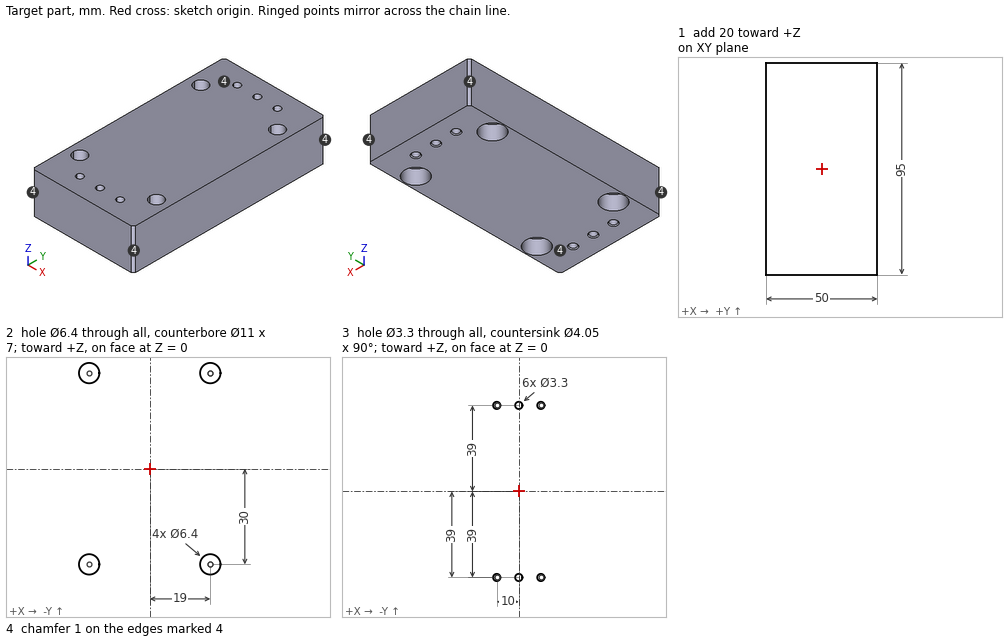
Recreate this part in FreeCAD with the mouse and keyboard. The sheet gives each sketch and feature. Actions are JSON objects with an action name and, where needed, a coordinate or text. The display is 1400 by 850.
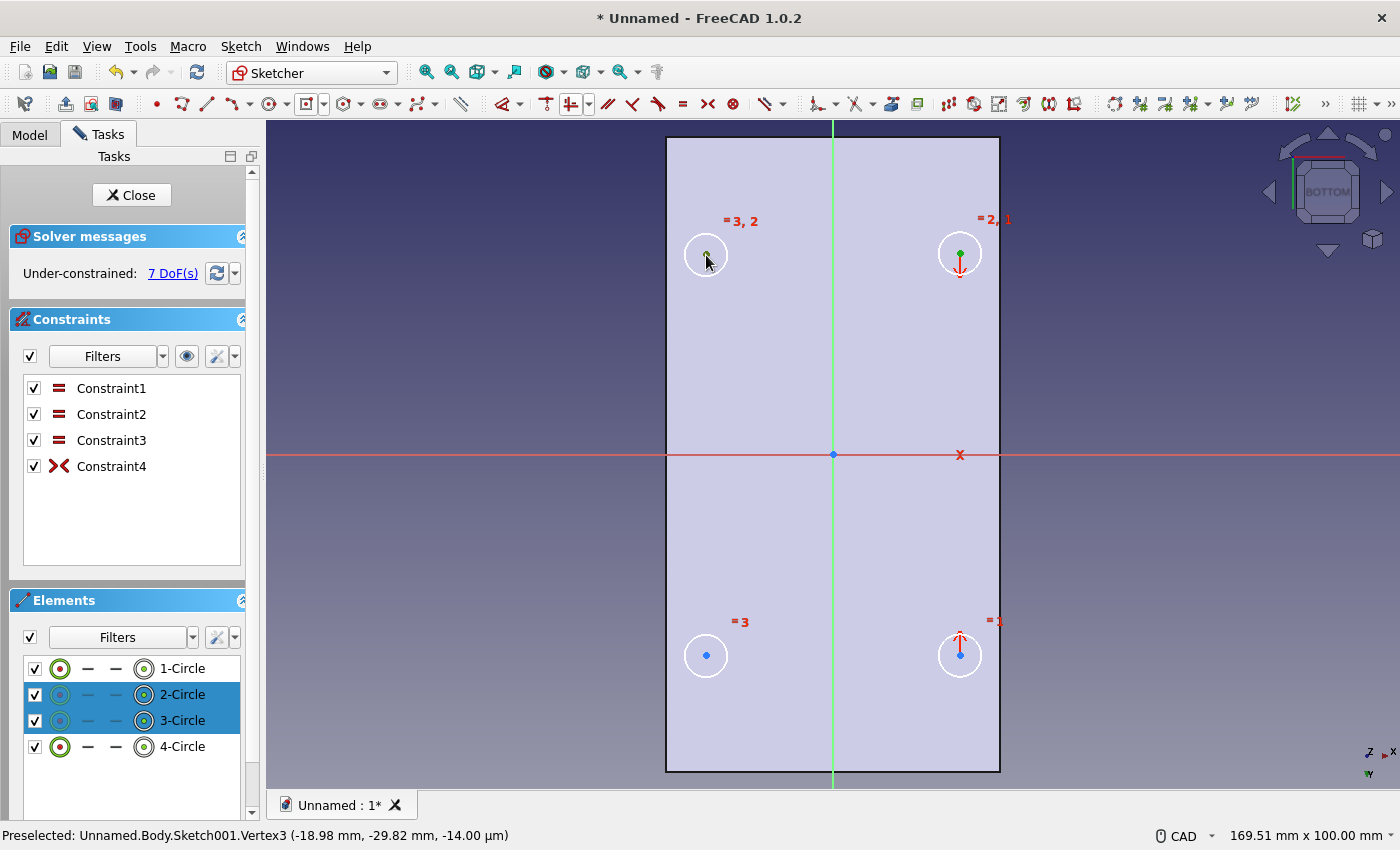
{"action": "left_click", "coordinate": [833, 717]}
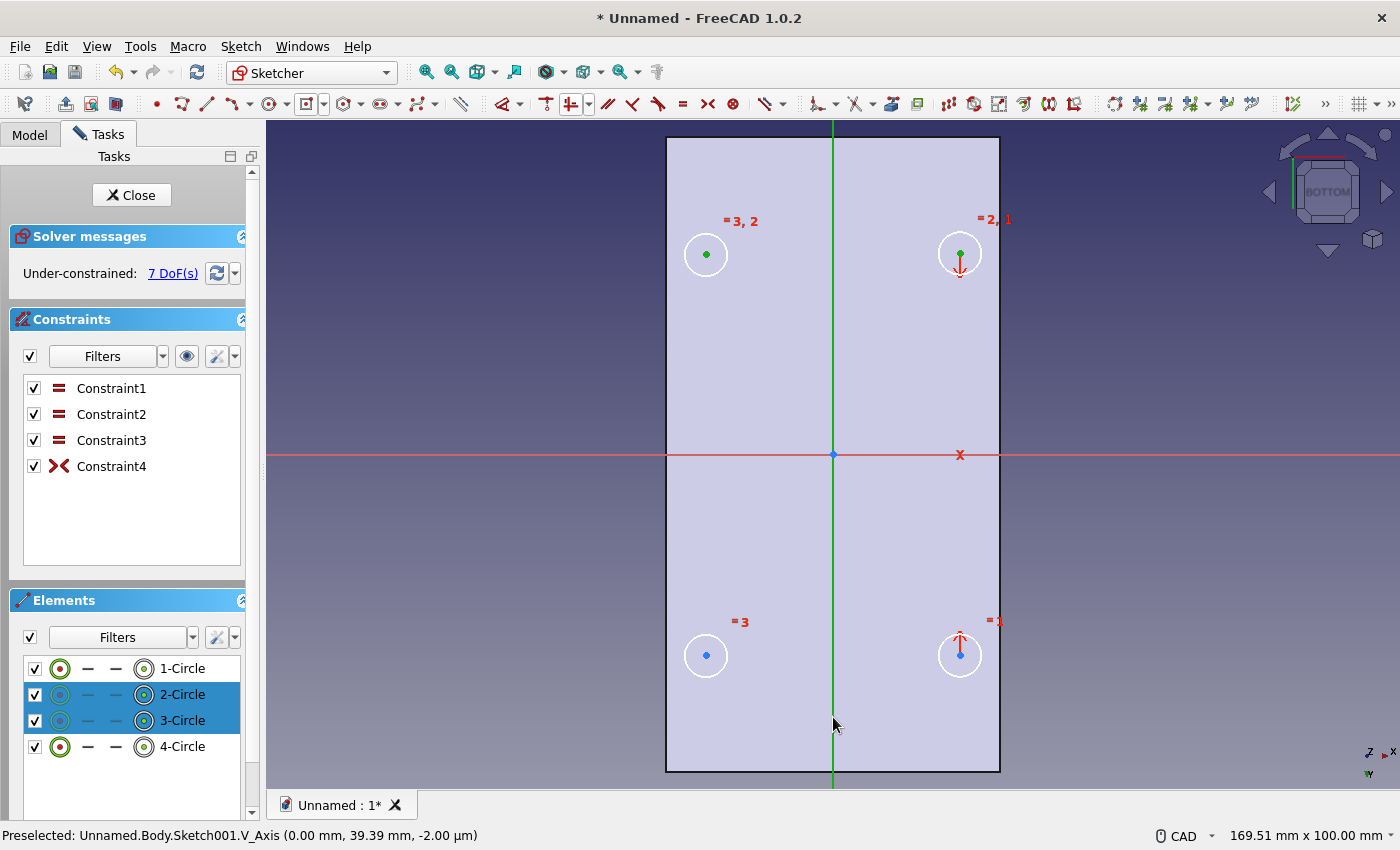
{"action": "left_click", "coordinate": [708, 104]}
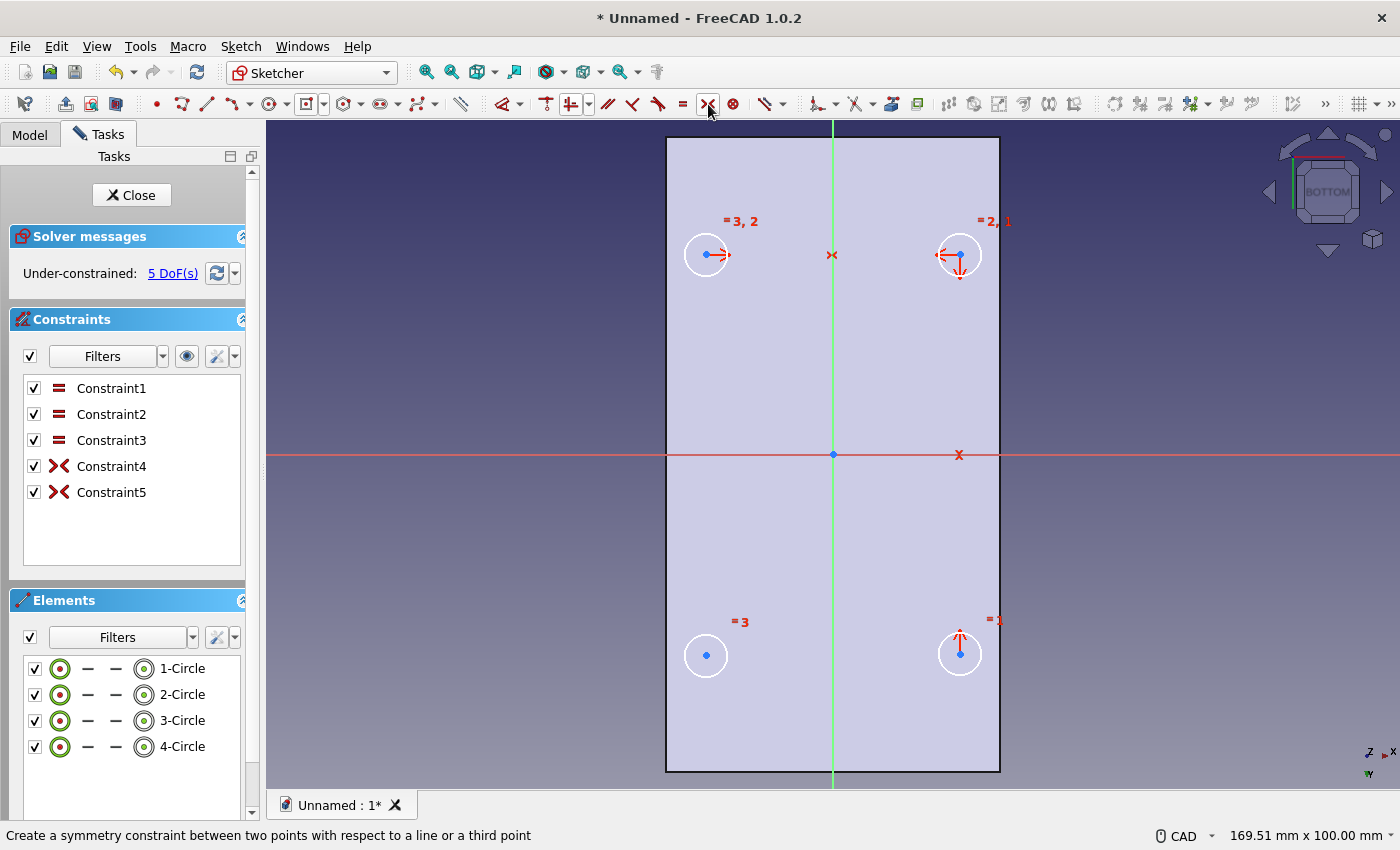
{"action": "left_click", "coordinate": [960, 654]}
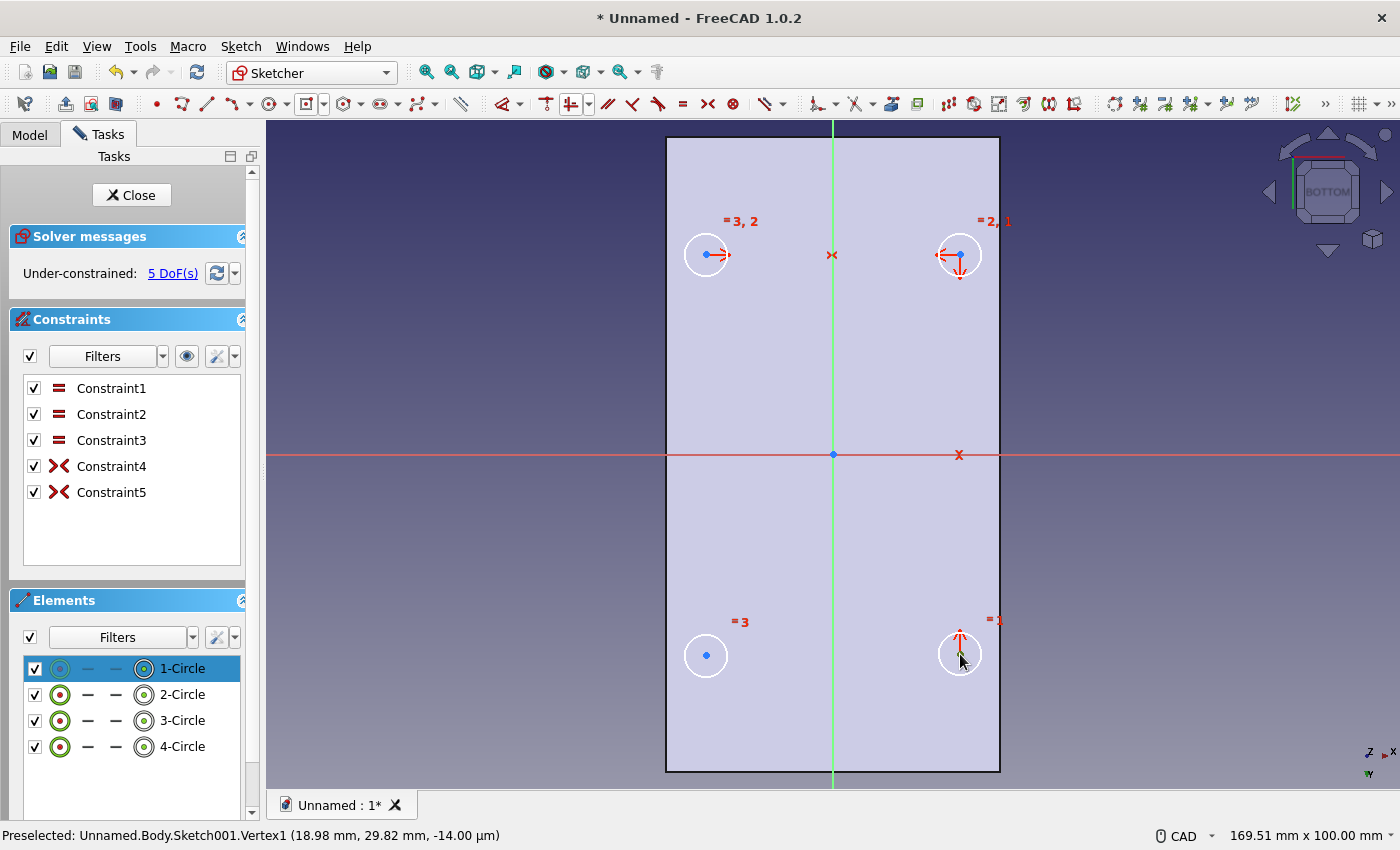
{"action": "left_click", "coordinate": [706, 656]}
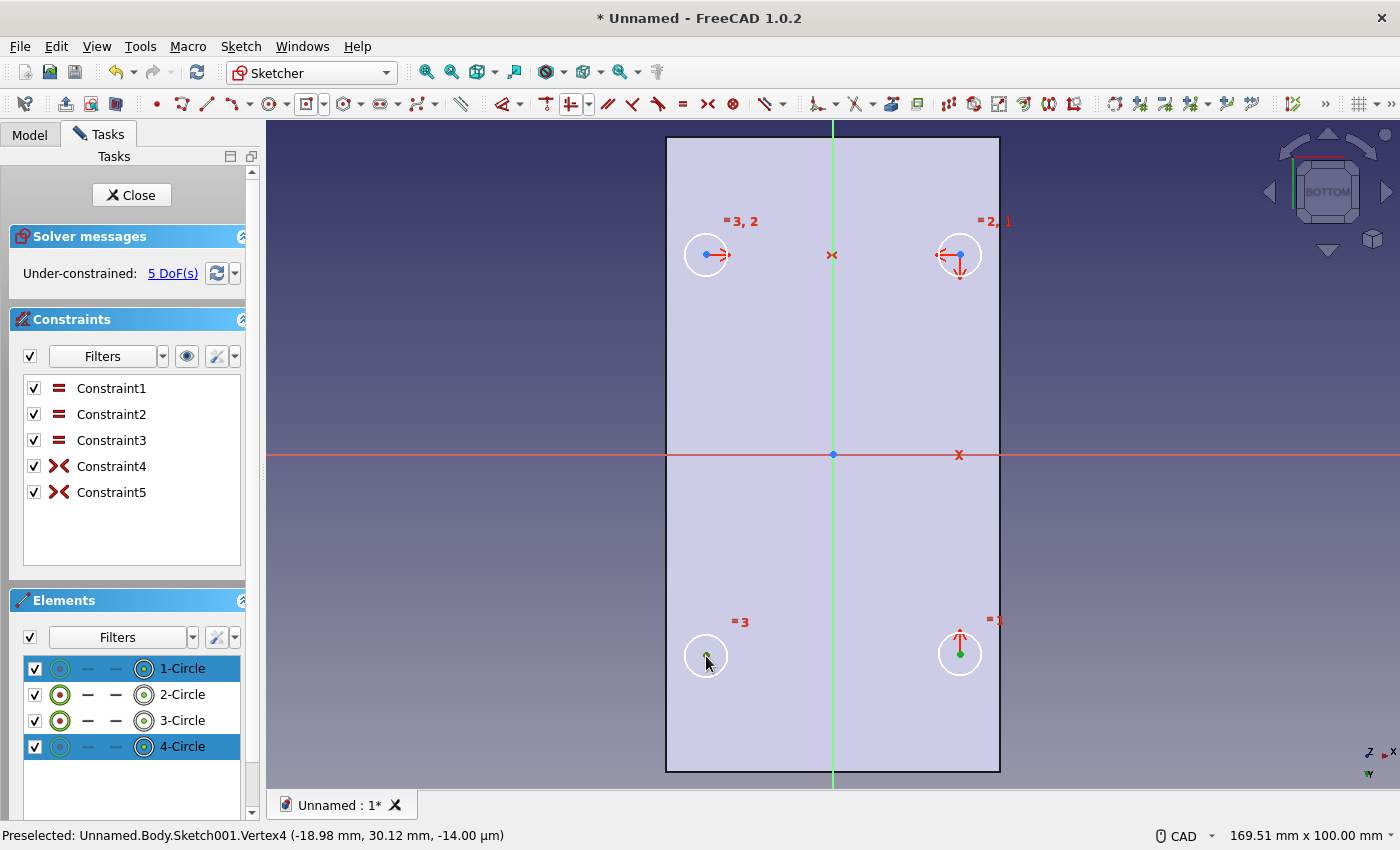
{"action": "left_click", "coordinate": [833, 717]}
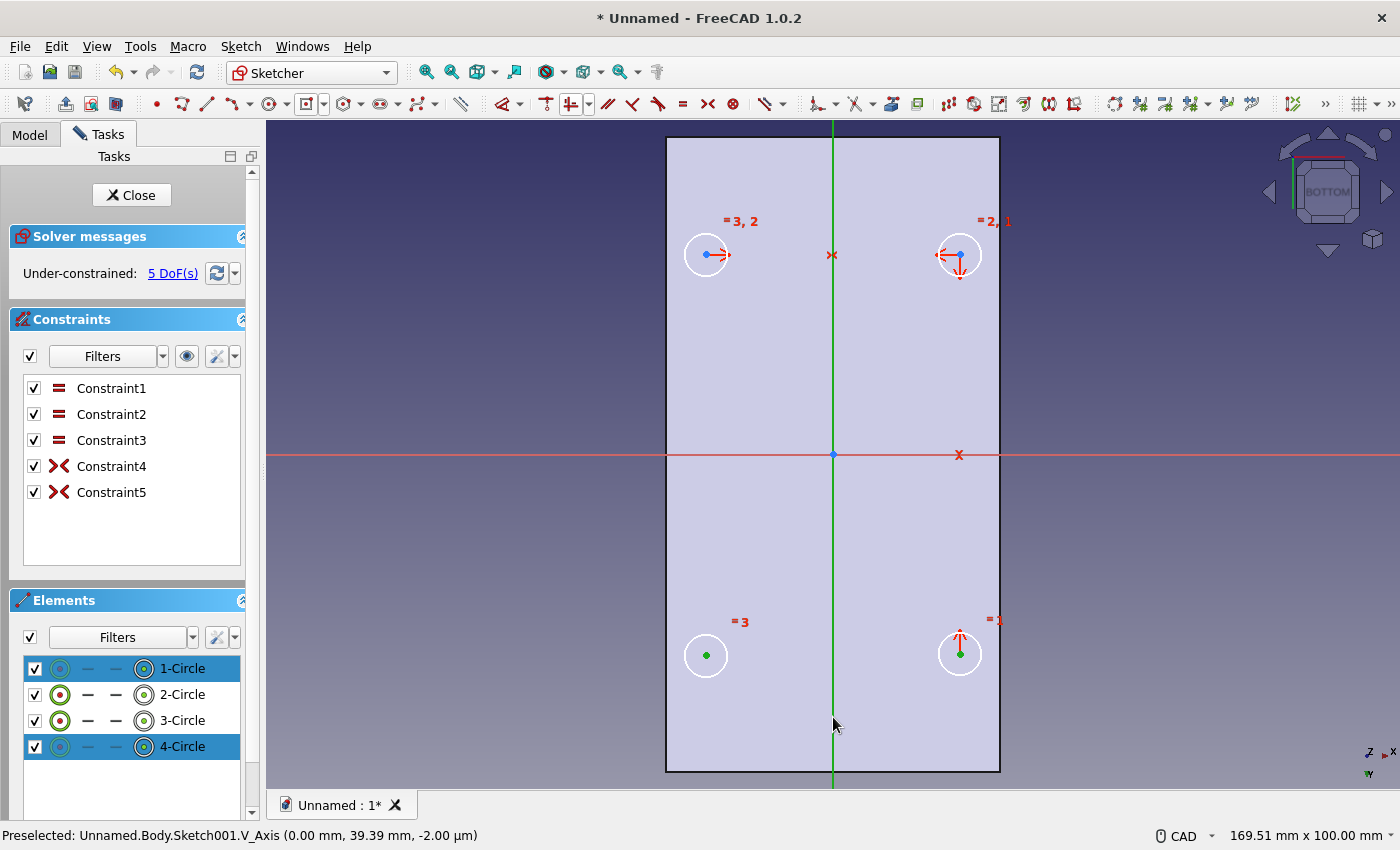
{"action": "left_click", "coordinate": [708, 104]}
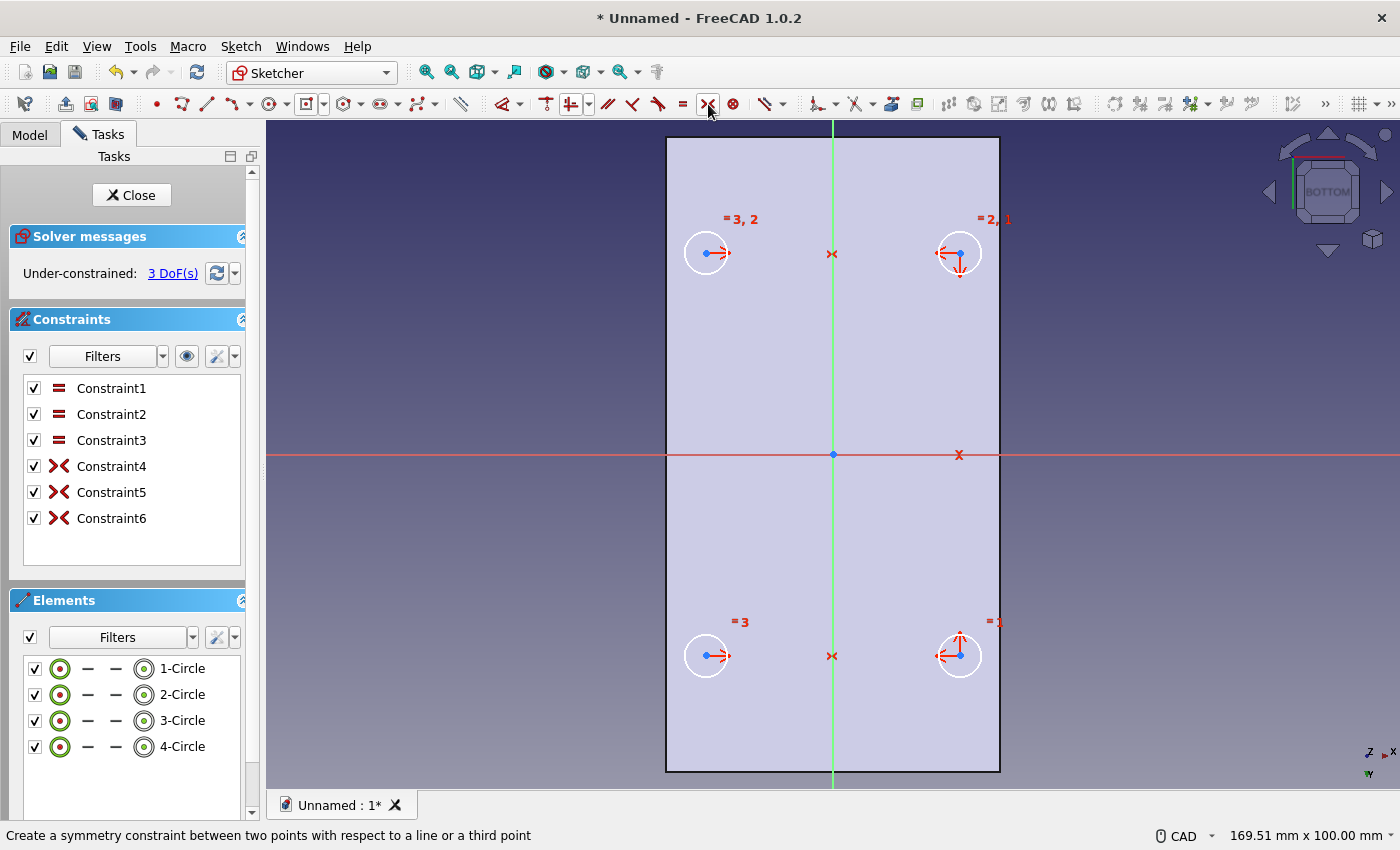
{"action": "left_click", "coordinate": [502, 104]}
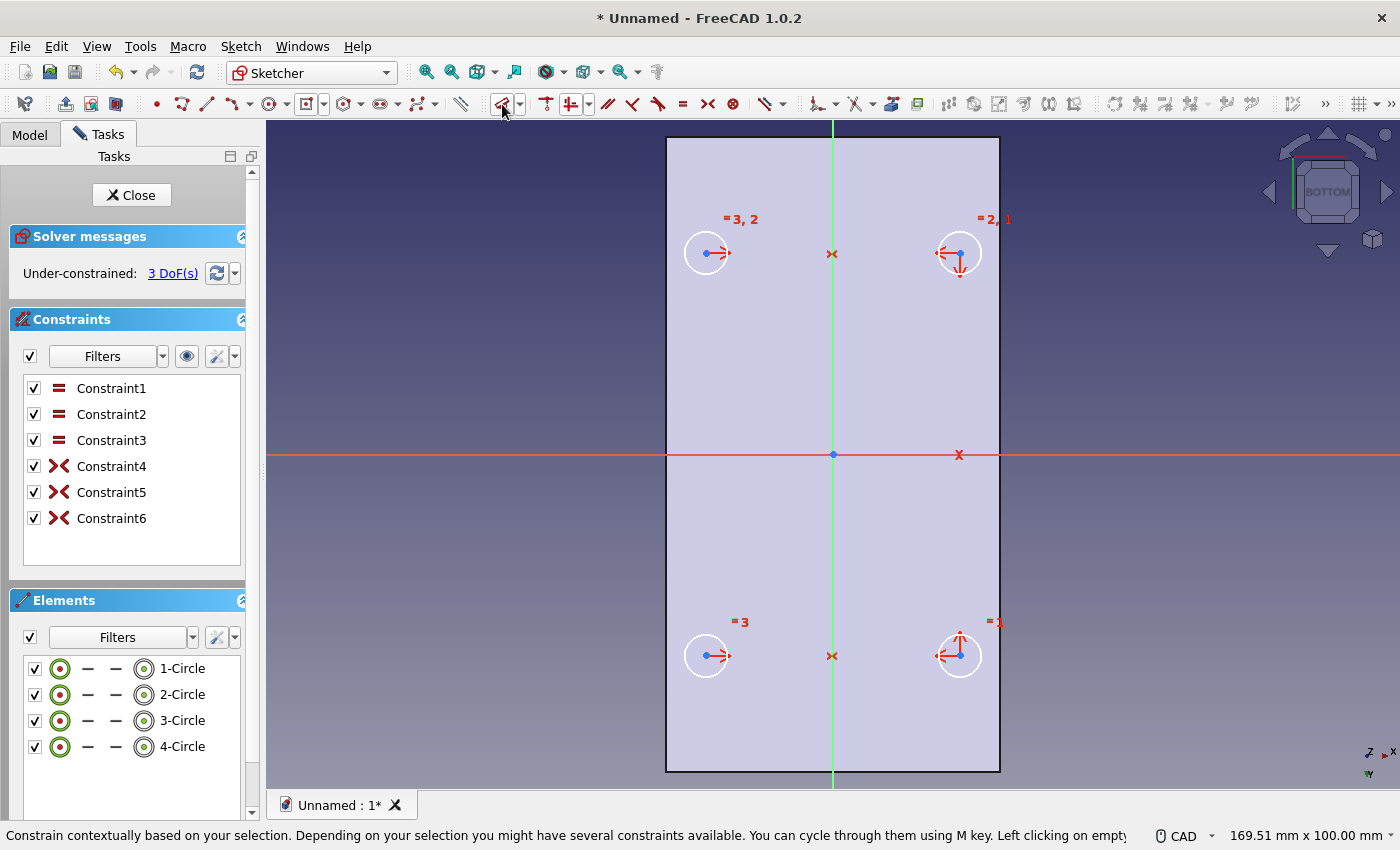
{"action": "left_click", "coordinate": [975, 641]}
{"action": "left_click", "coordinate": [998, 618]}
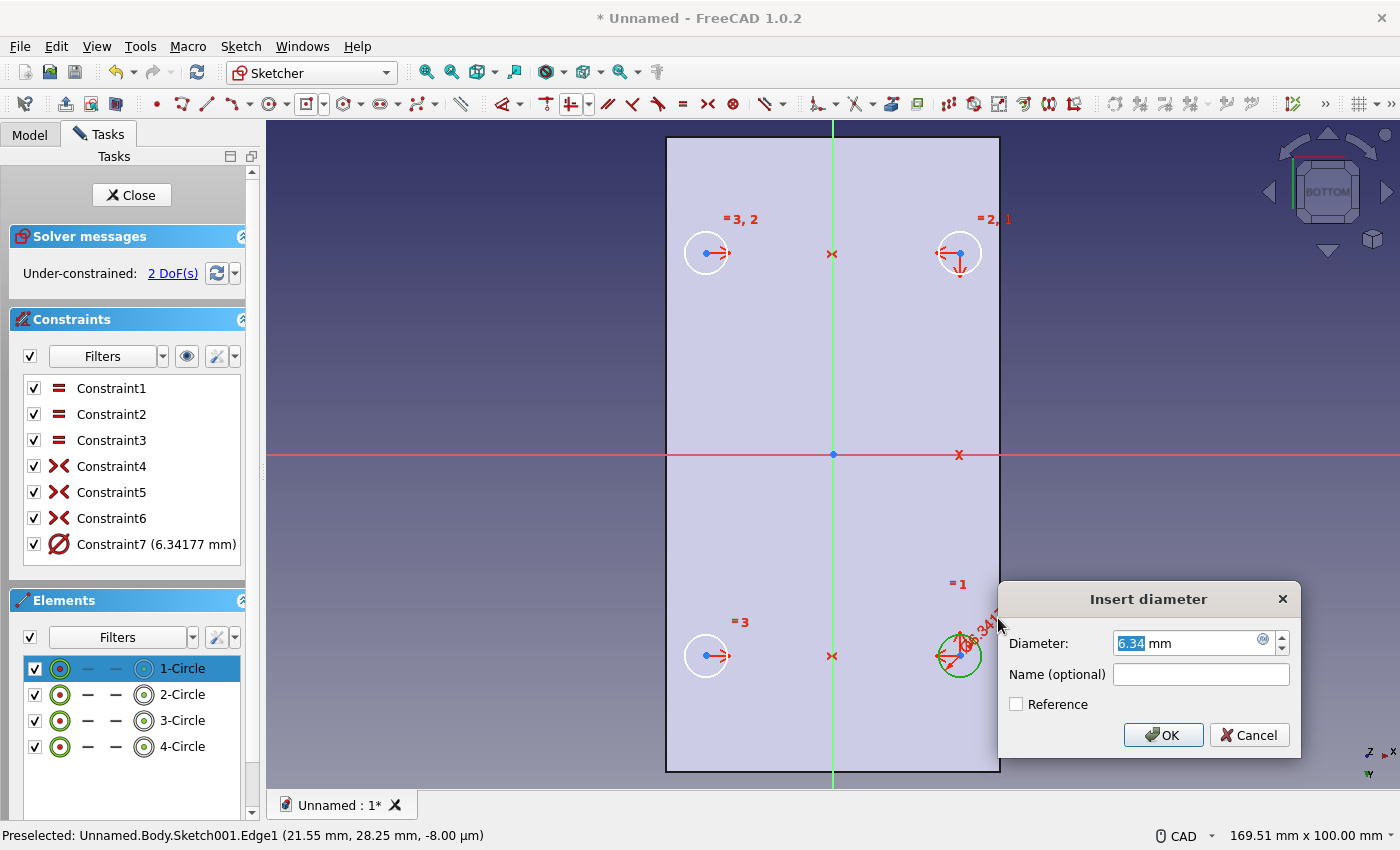
{"action": "type", "text": "6.4"}
{"action": "key", "text": "Return"}